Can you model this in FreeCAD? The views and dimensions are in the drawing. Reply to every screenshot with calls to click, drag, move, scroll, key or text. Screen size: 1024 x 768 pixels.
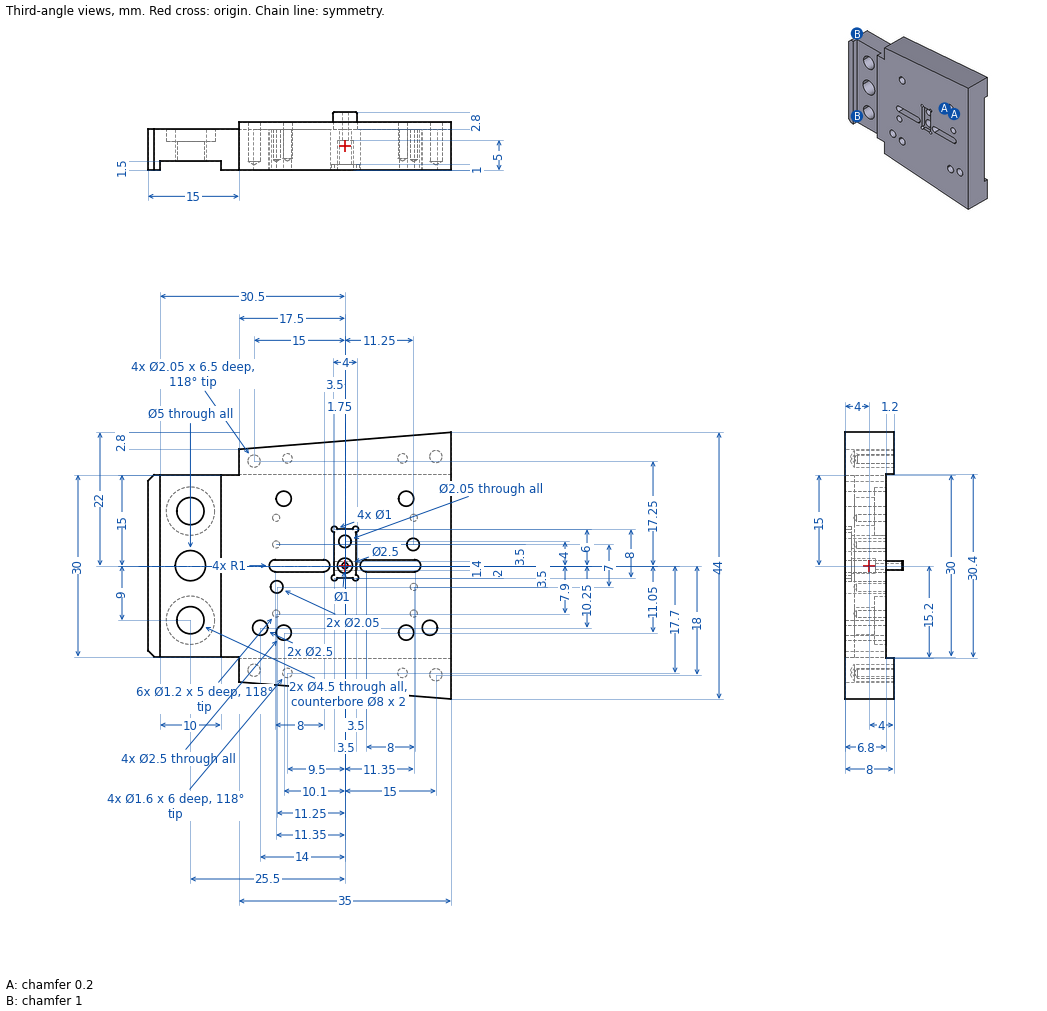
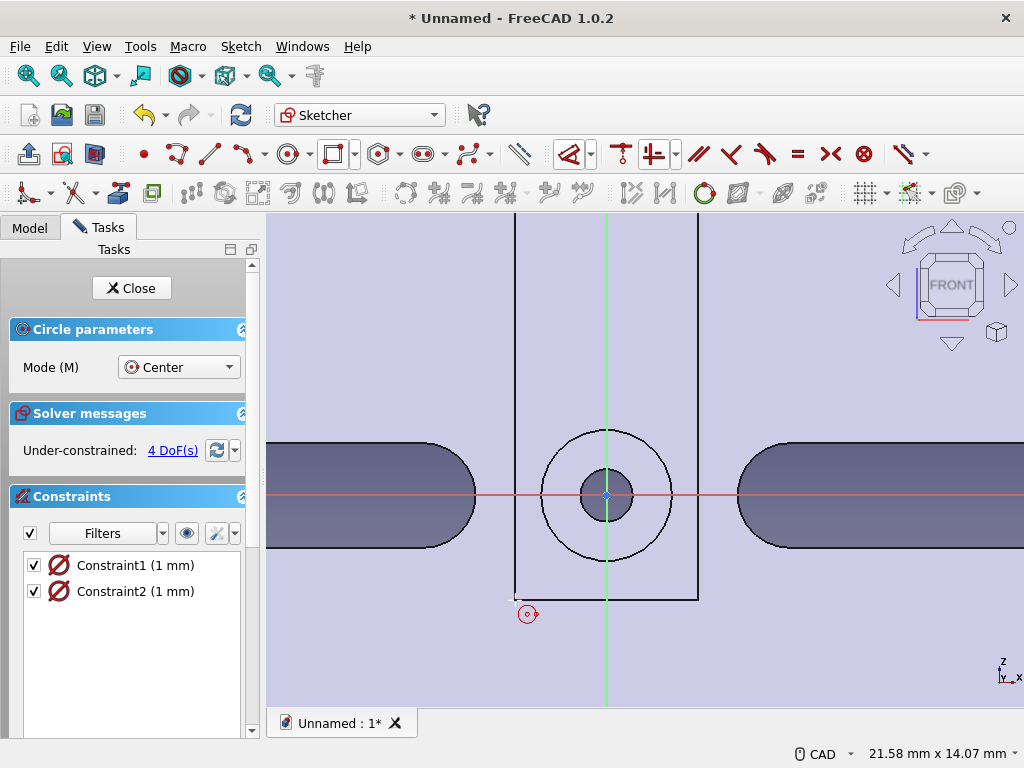
click(515, 600)
move(533, 582)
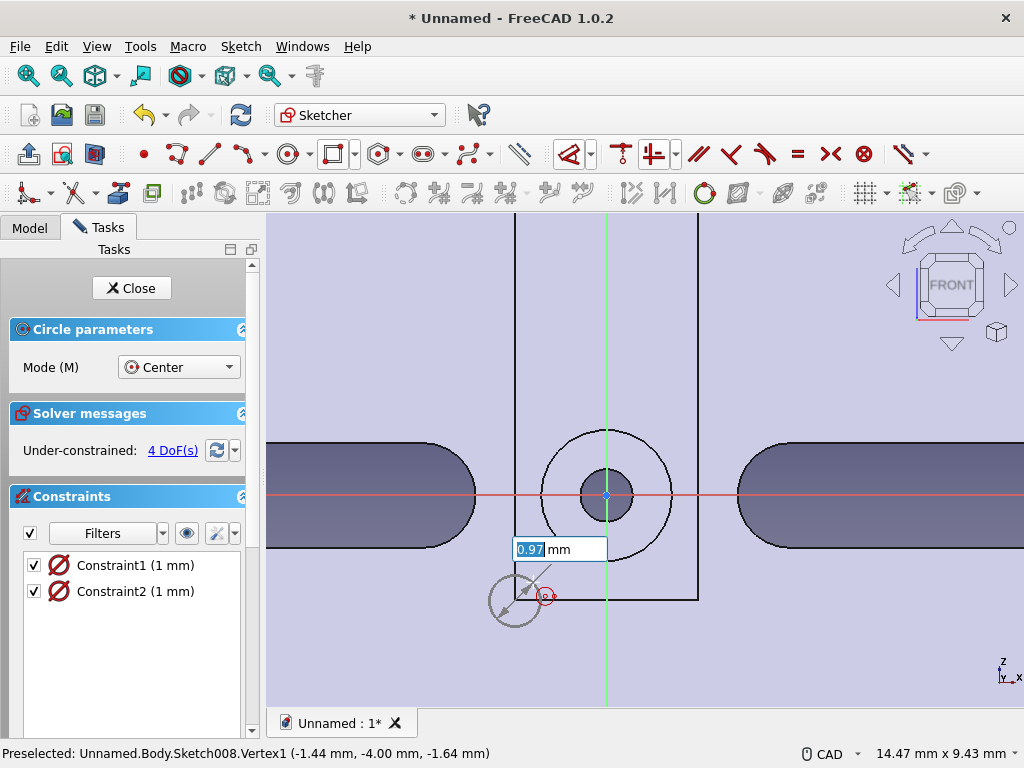
text(1)
key(Return)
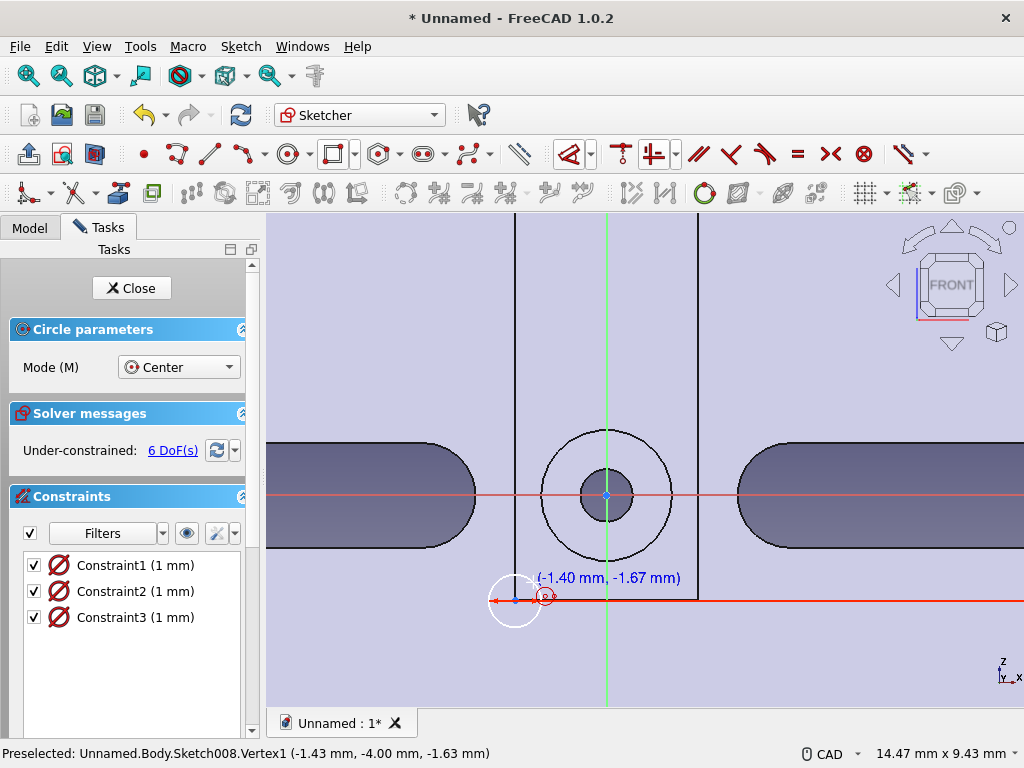
click(698, 600)
move(717, 582)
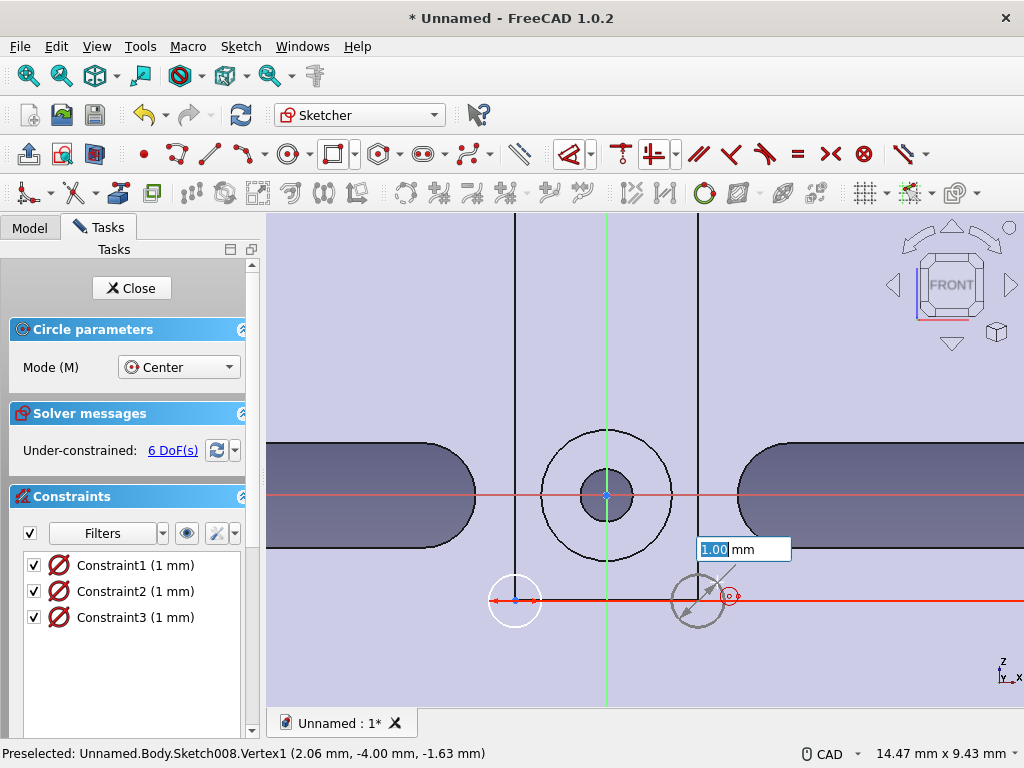
text(1)
key(Return)
key(Escape)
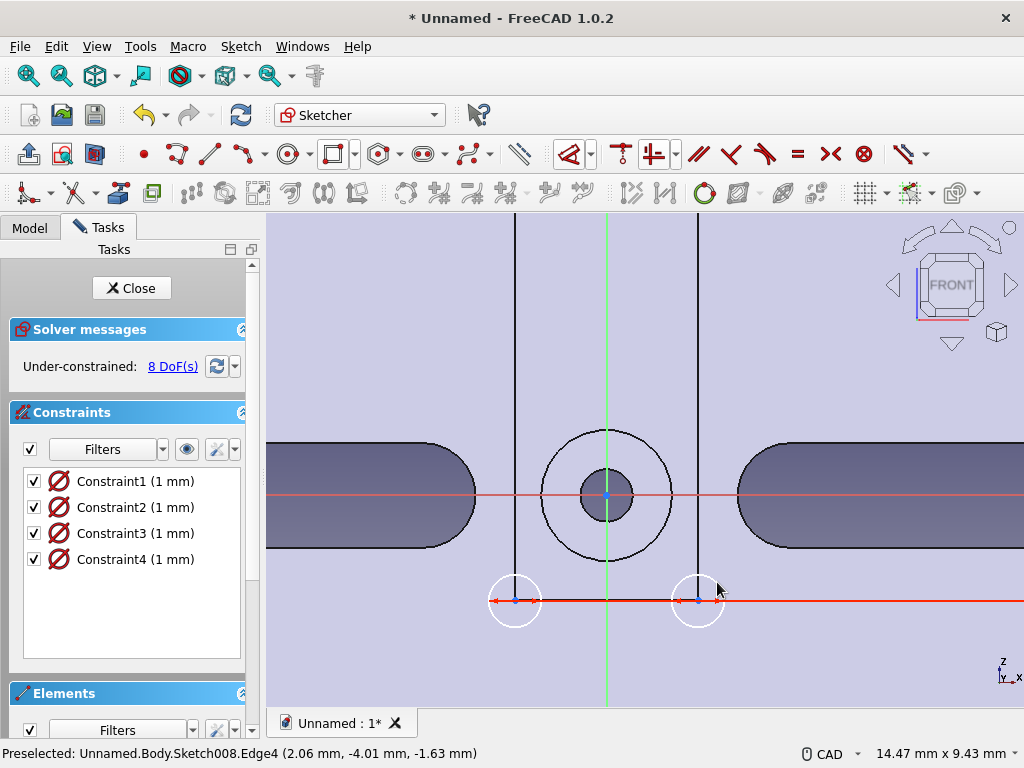
scroll(515, 601, down, 2)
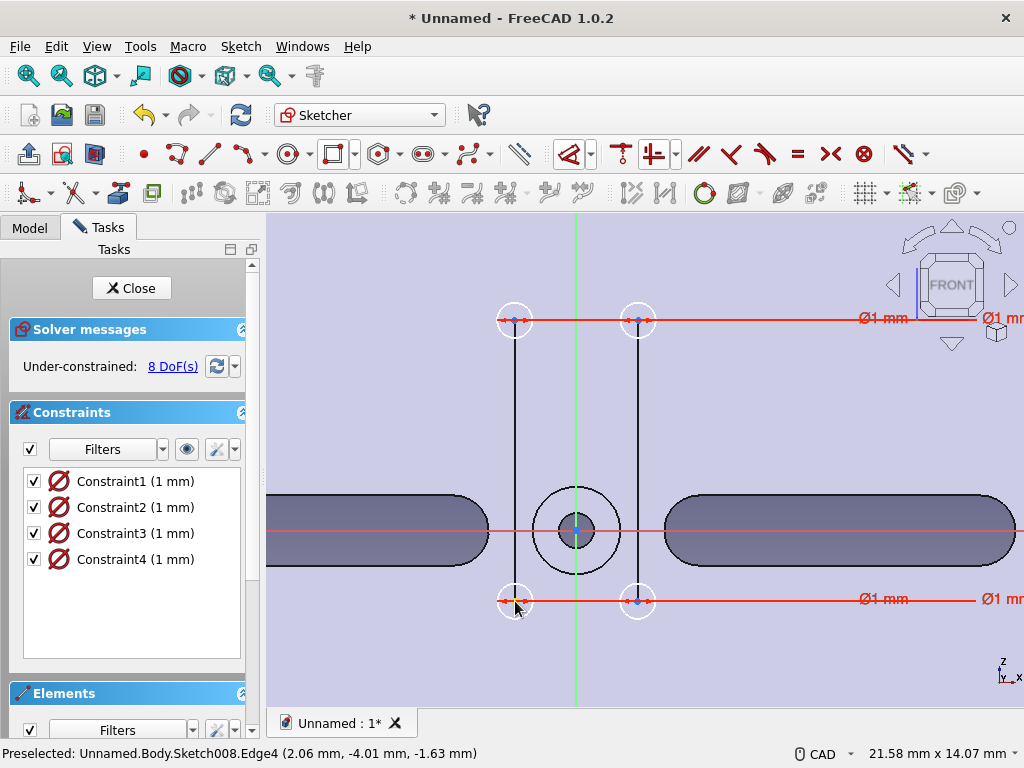
click(515, 320)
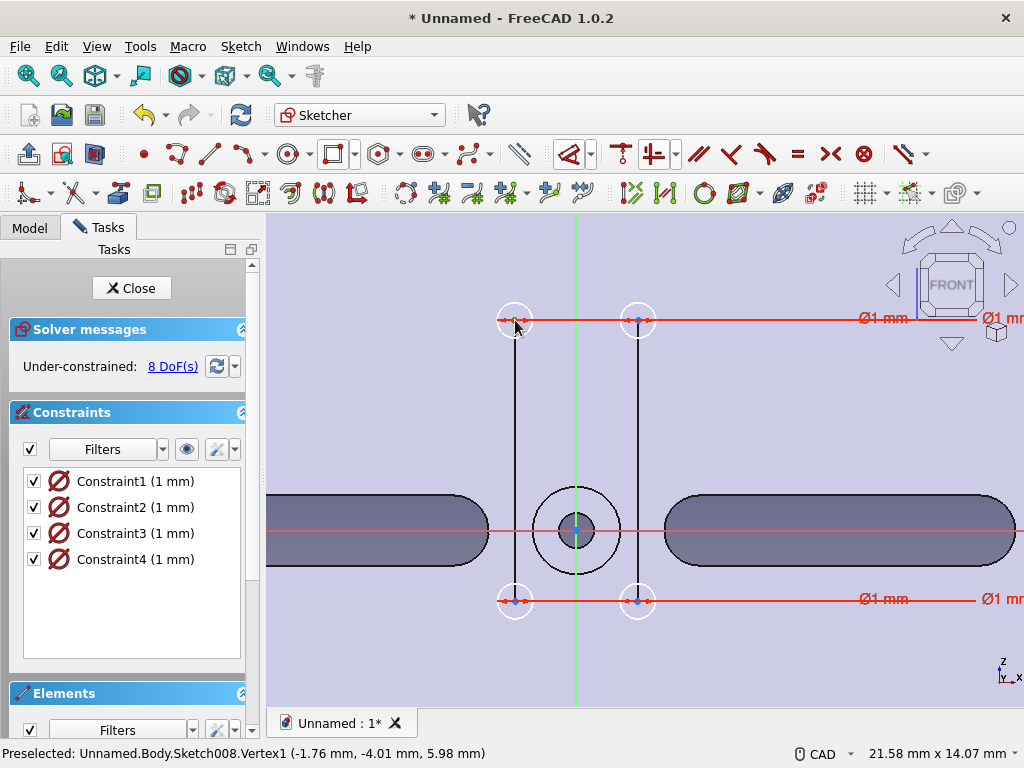
click(638, 320)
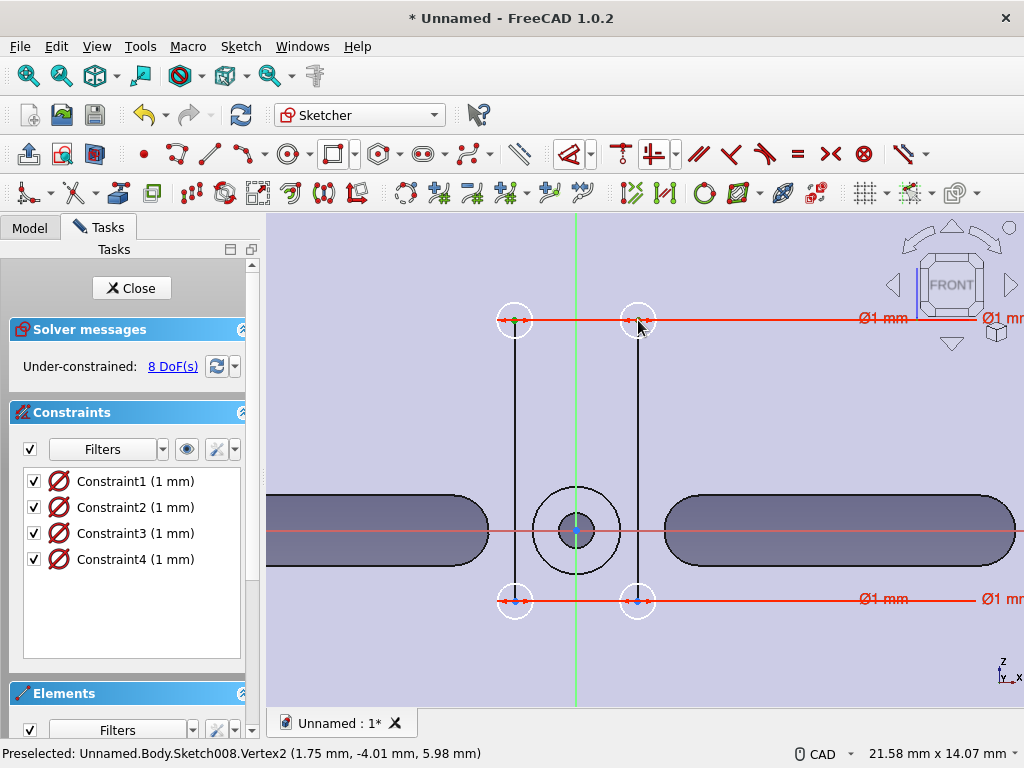
click(576, 648)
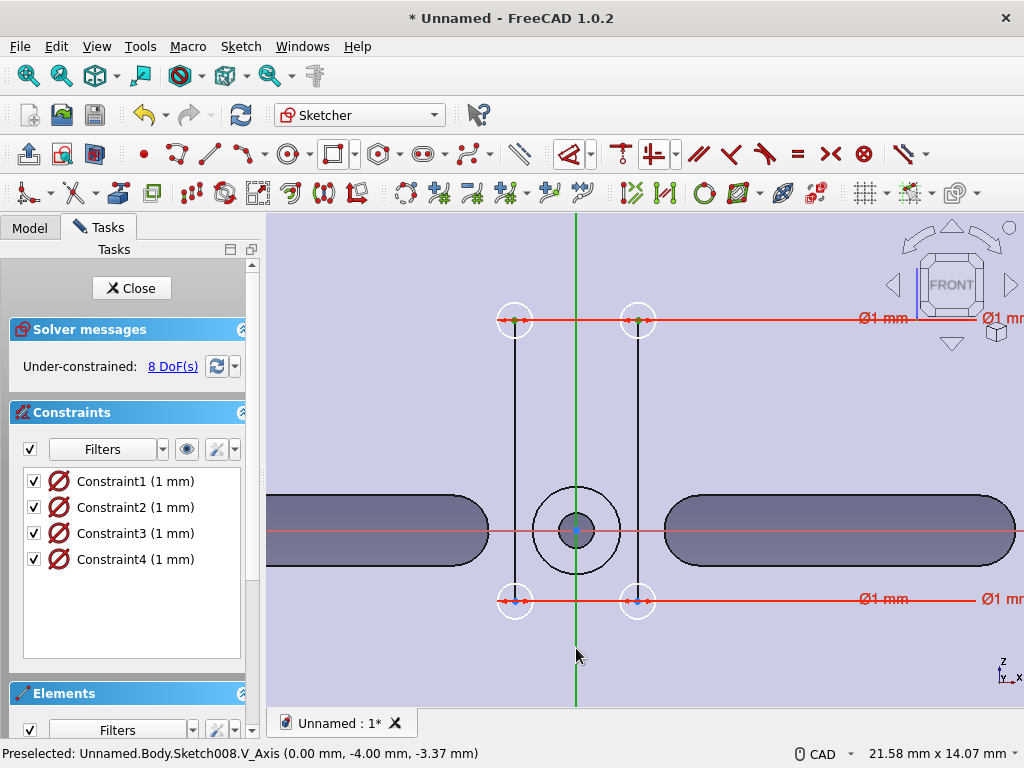
click(831, 154)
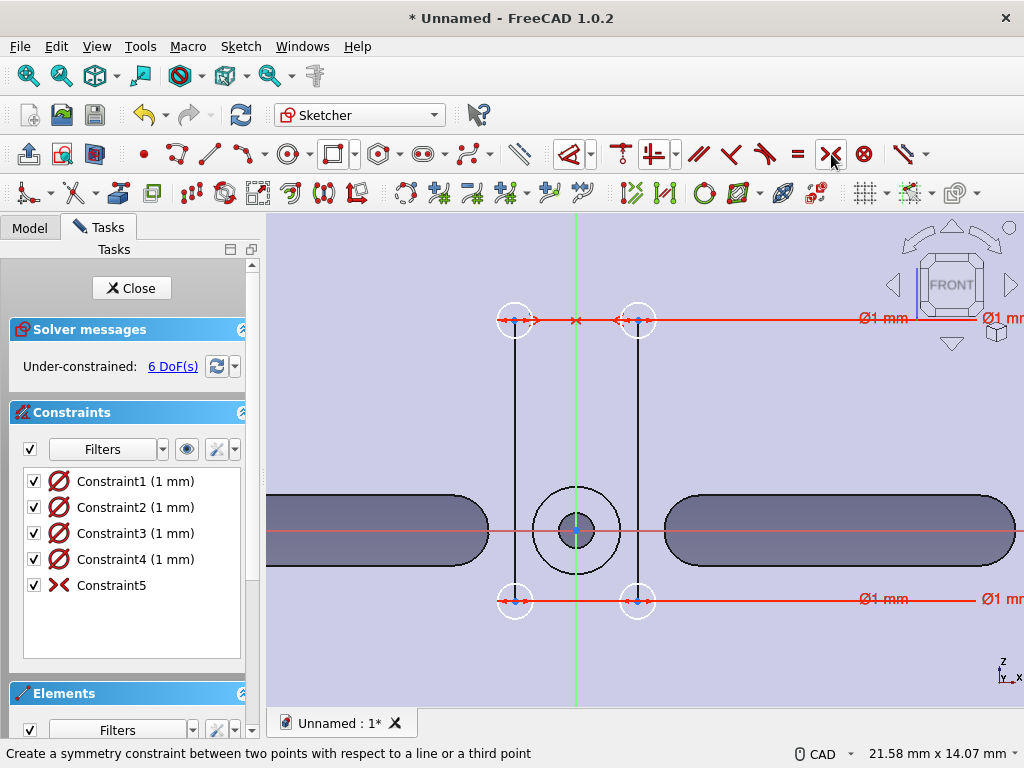
click(515, 601)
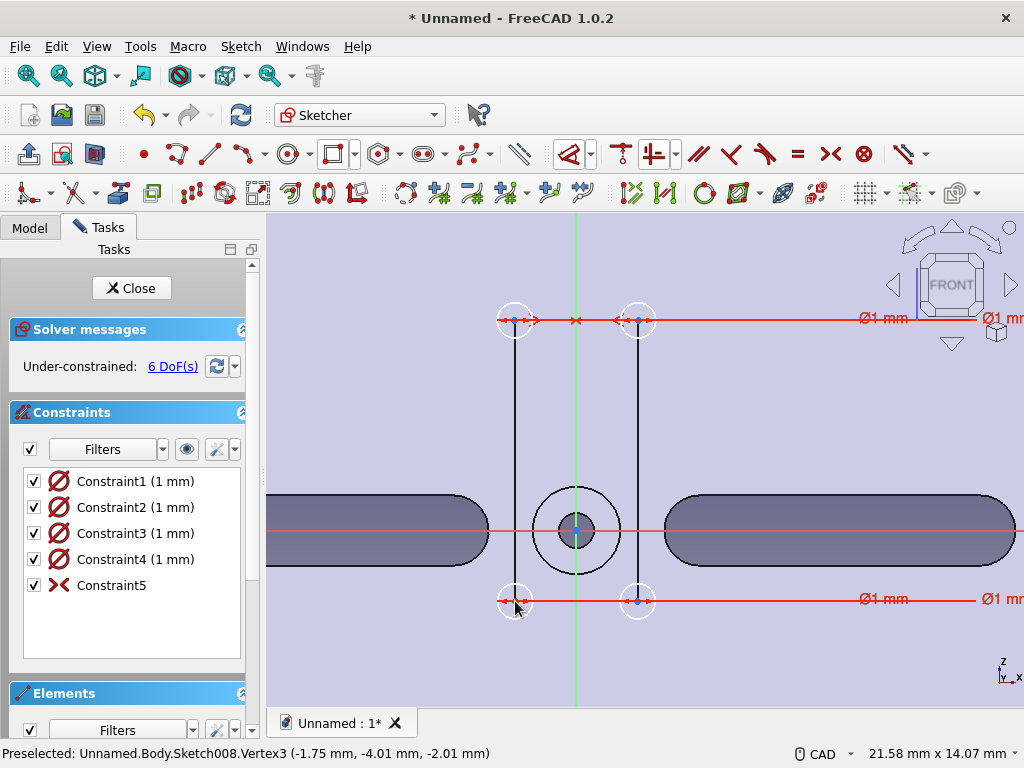
click(638, 601)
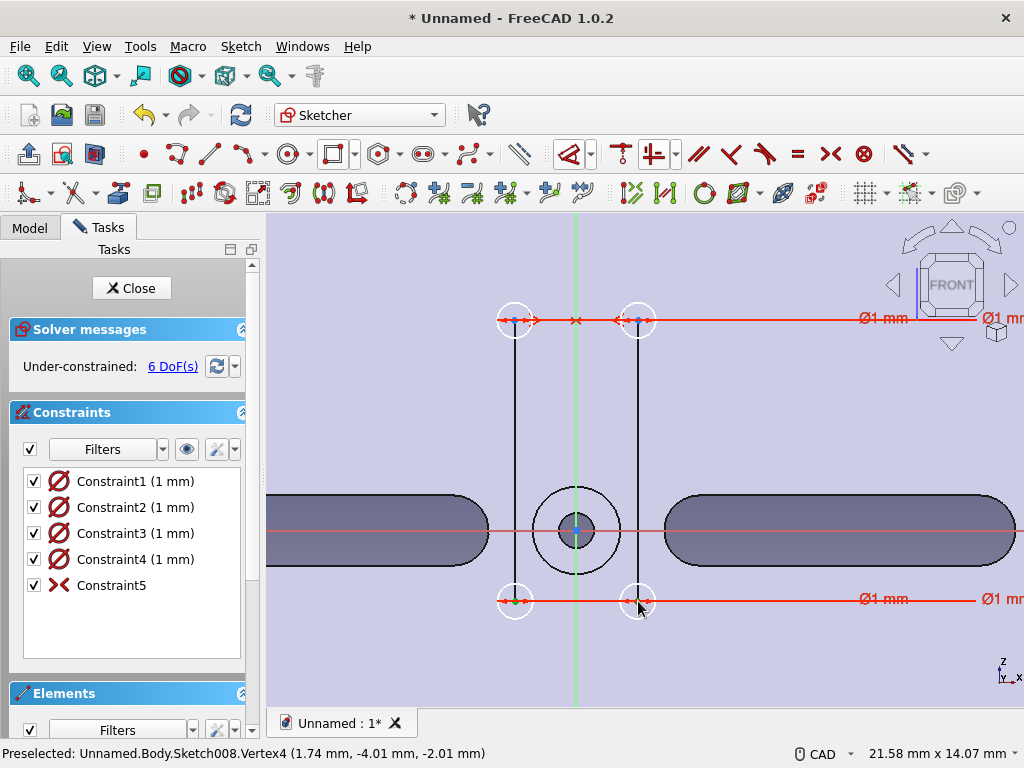
click(576, 648)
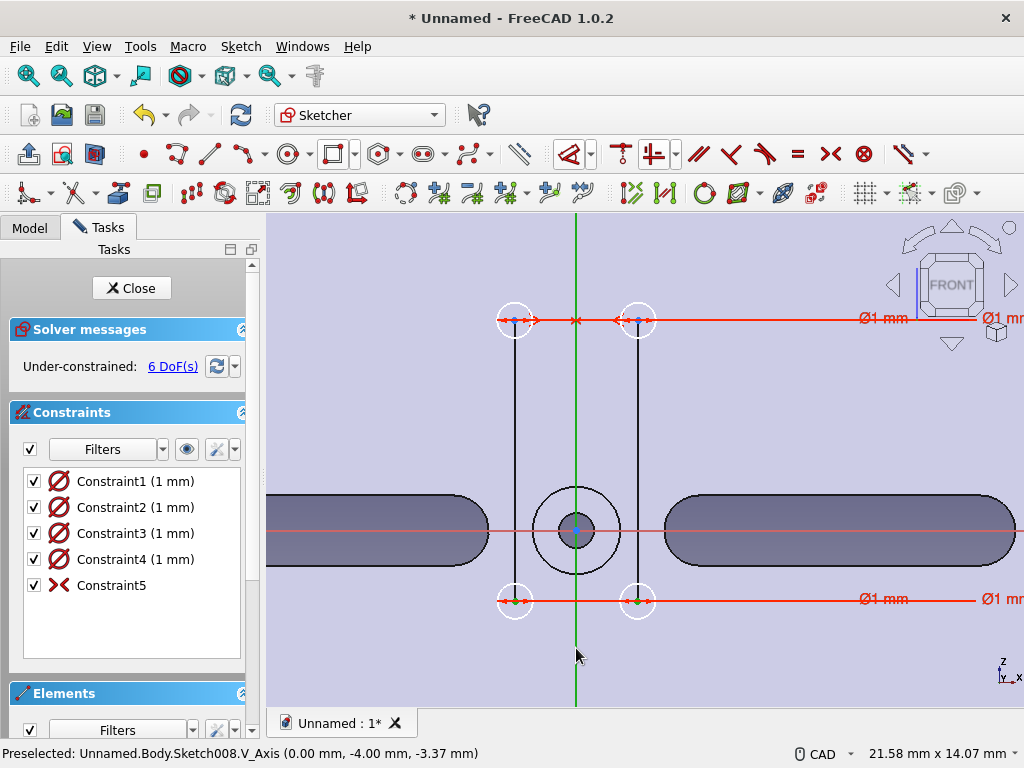
click(831, 154)